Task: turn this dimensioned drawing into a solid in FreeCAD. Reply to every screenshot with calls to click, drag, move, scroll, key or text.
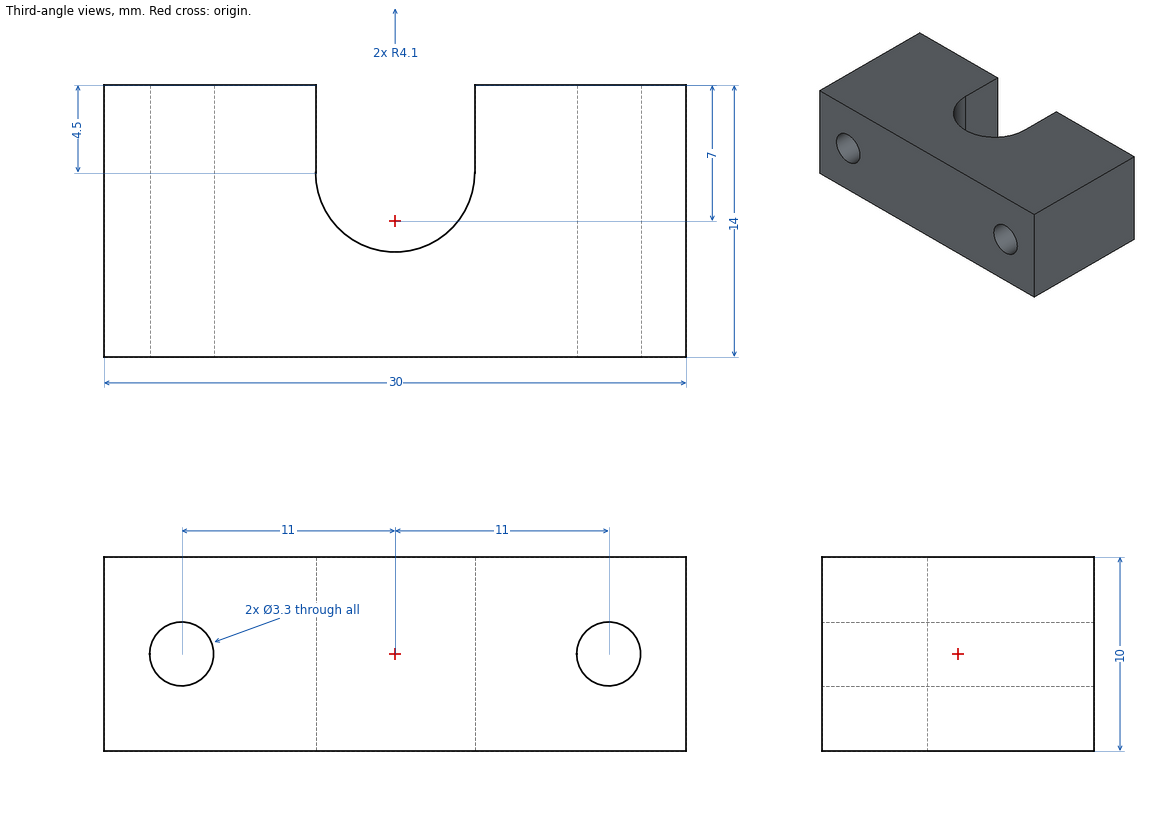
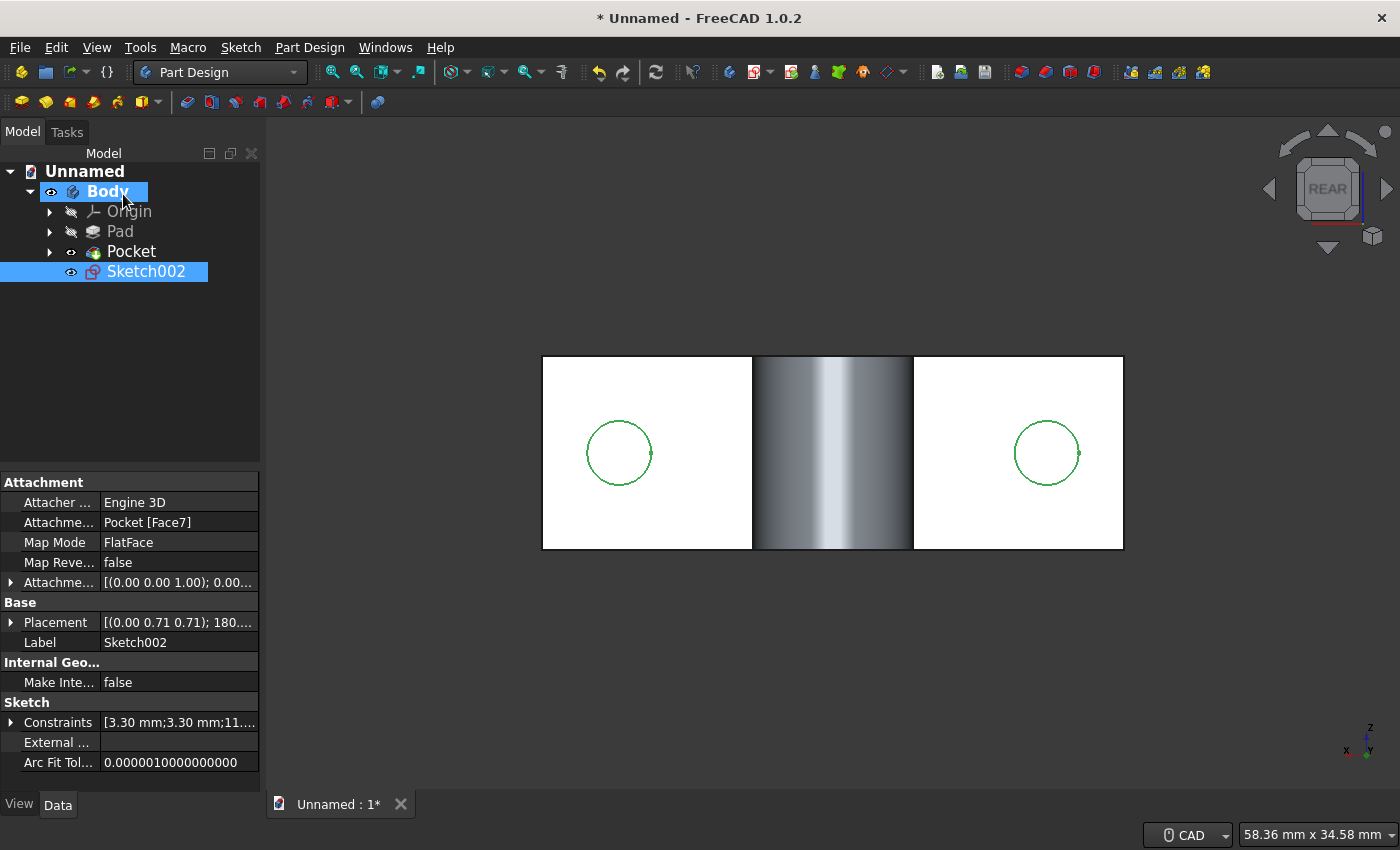
click(212, 102)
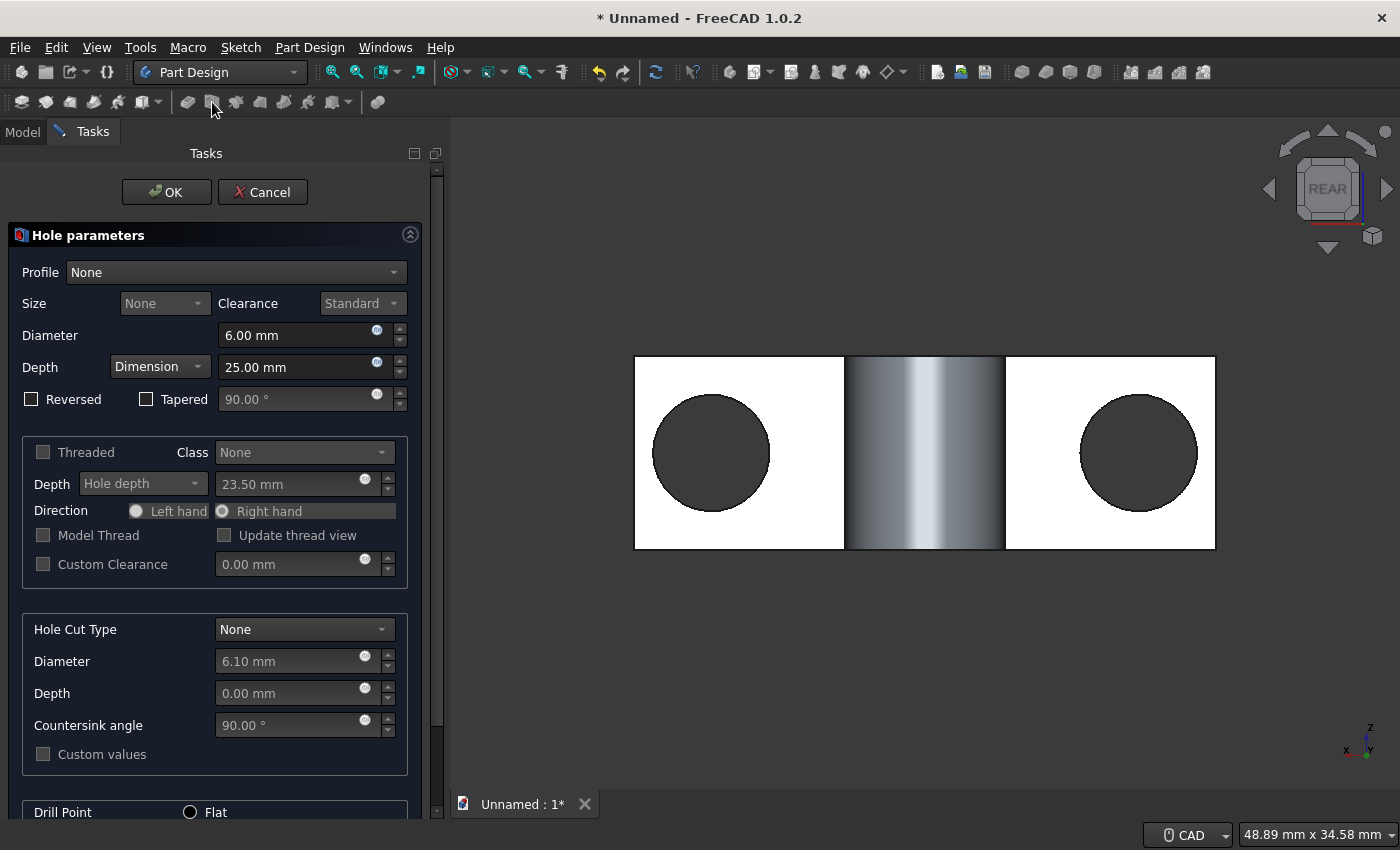
triple_click(305, 335)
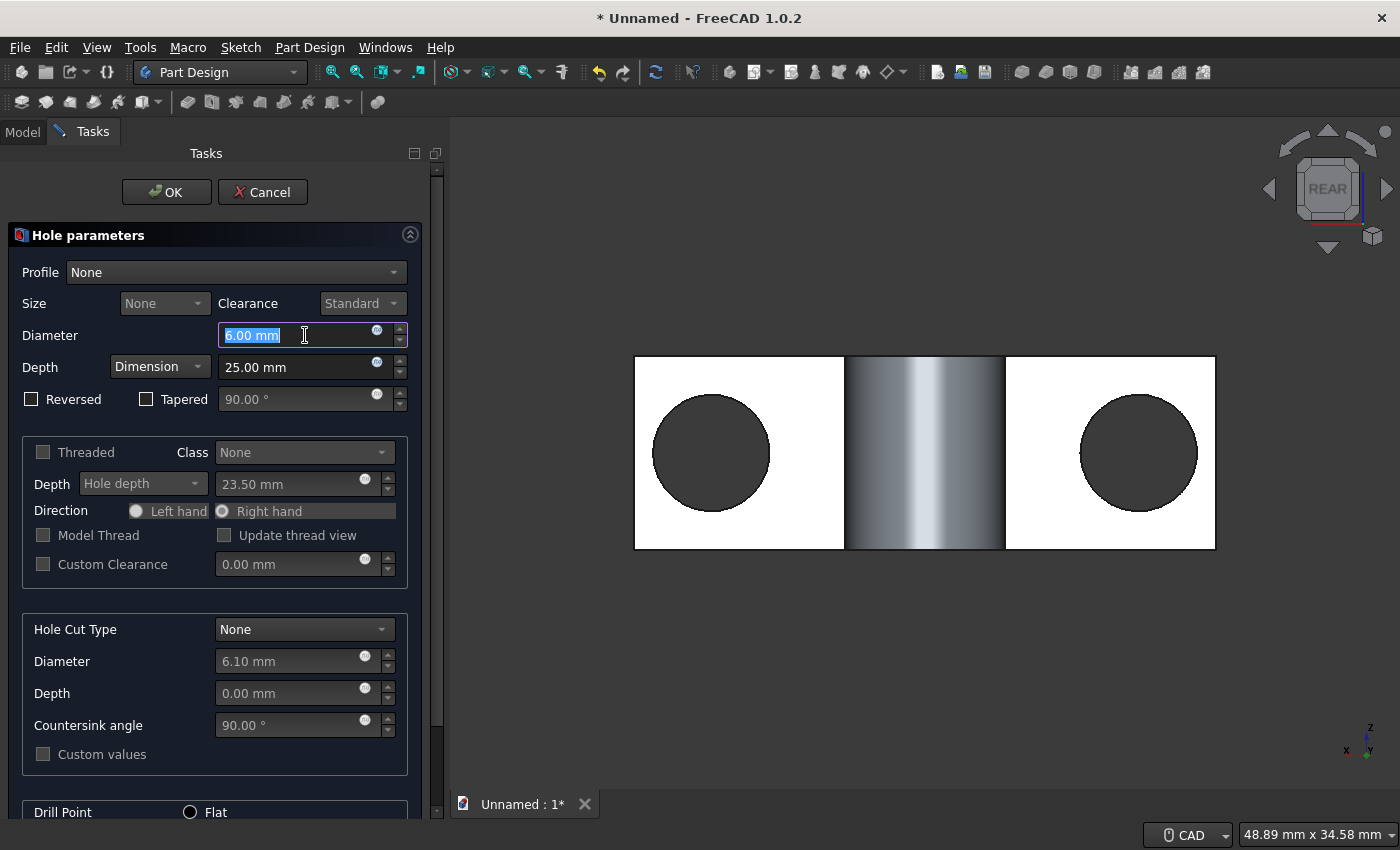
text(3.3)
key(Tab)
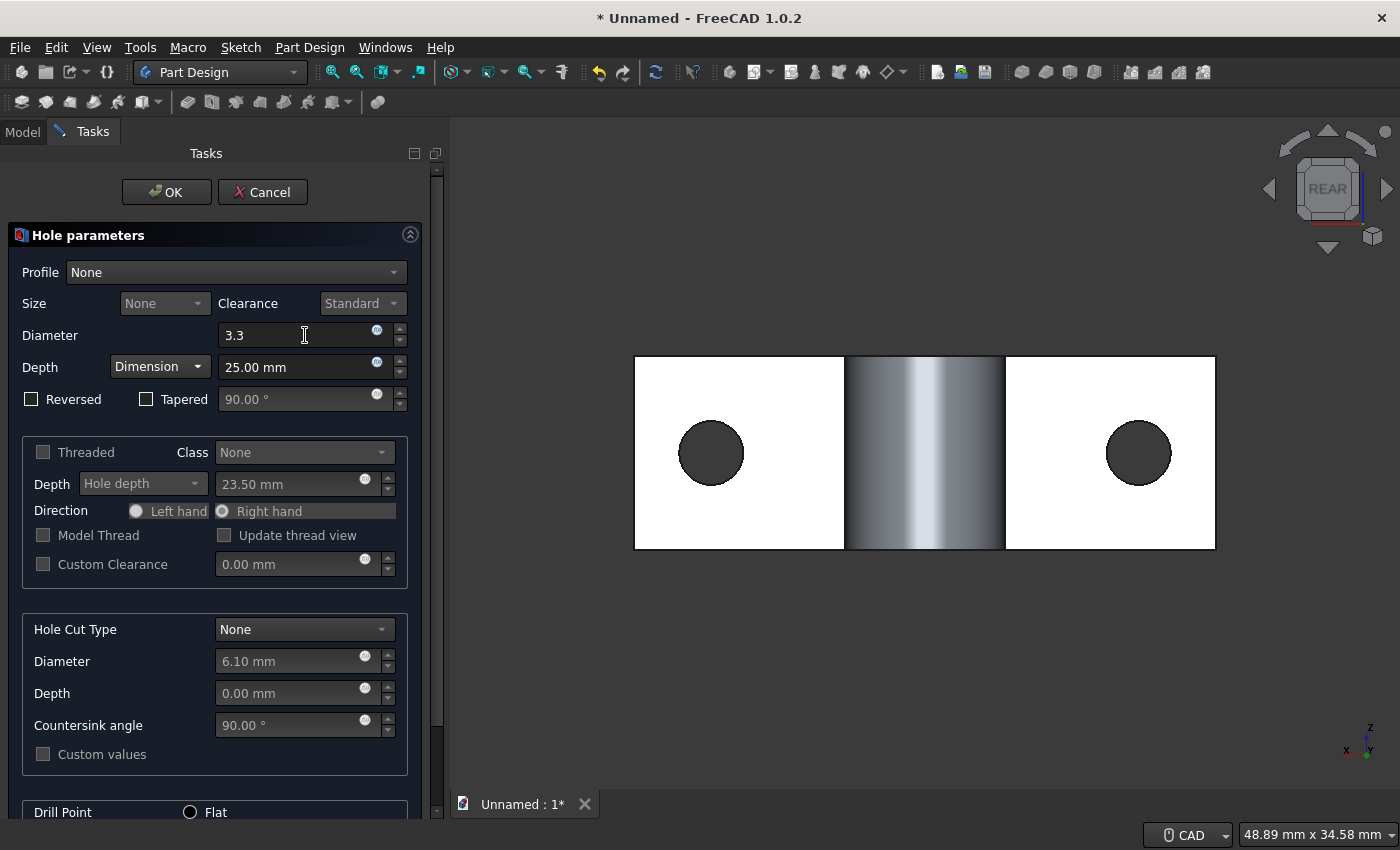
click(161, 366)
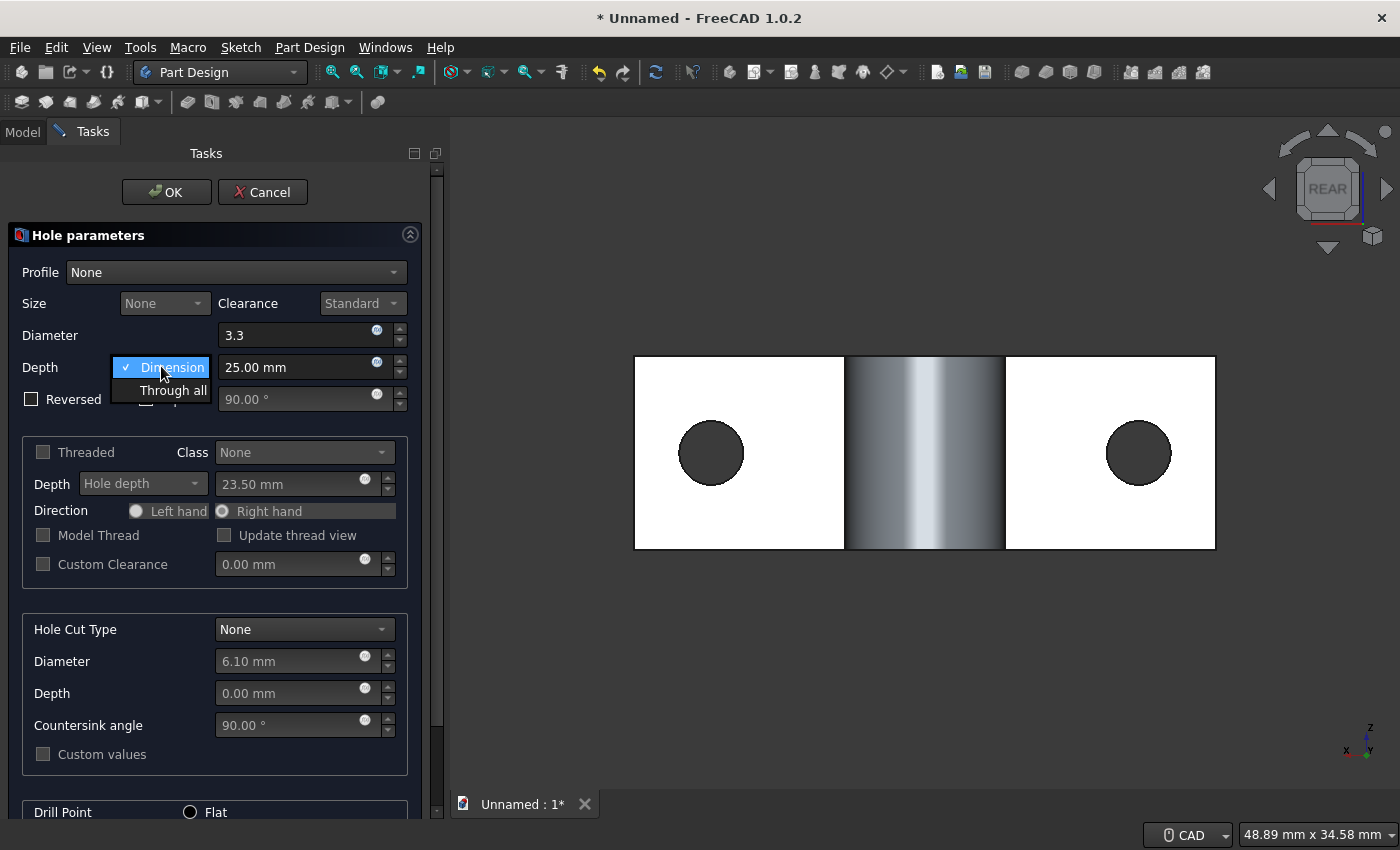
click(160, 390)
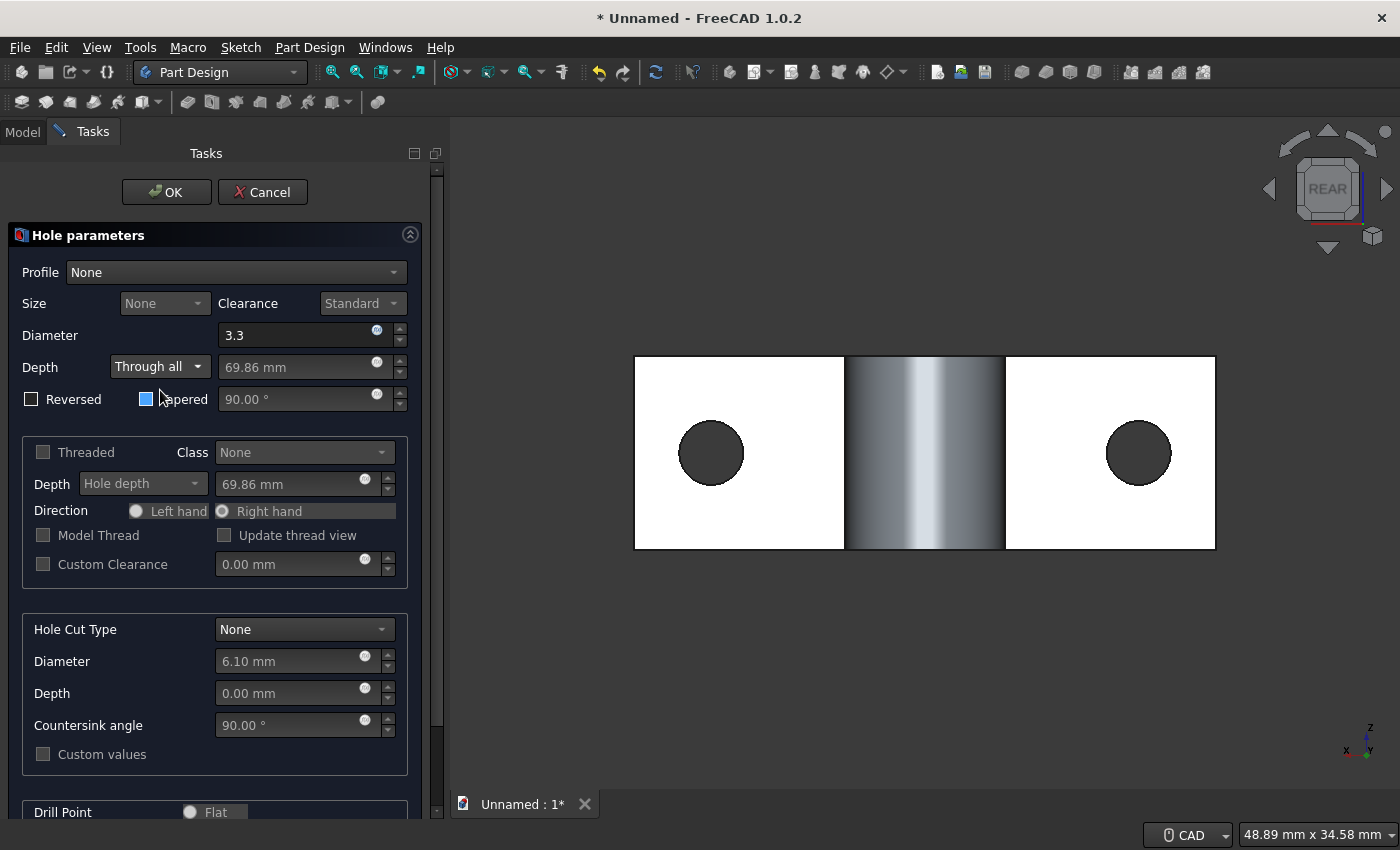
click(167, 192)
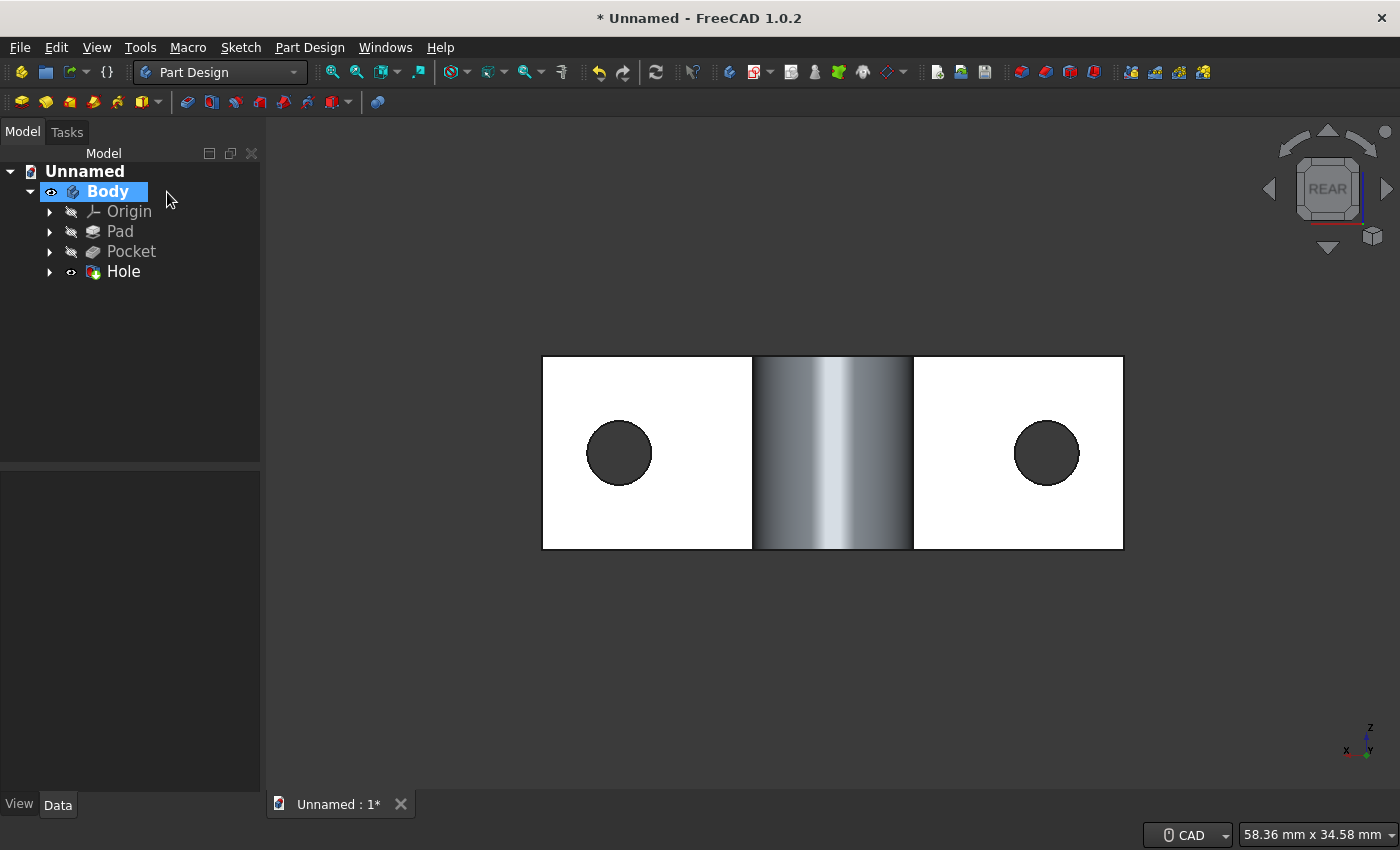
key(0)